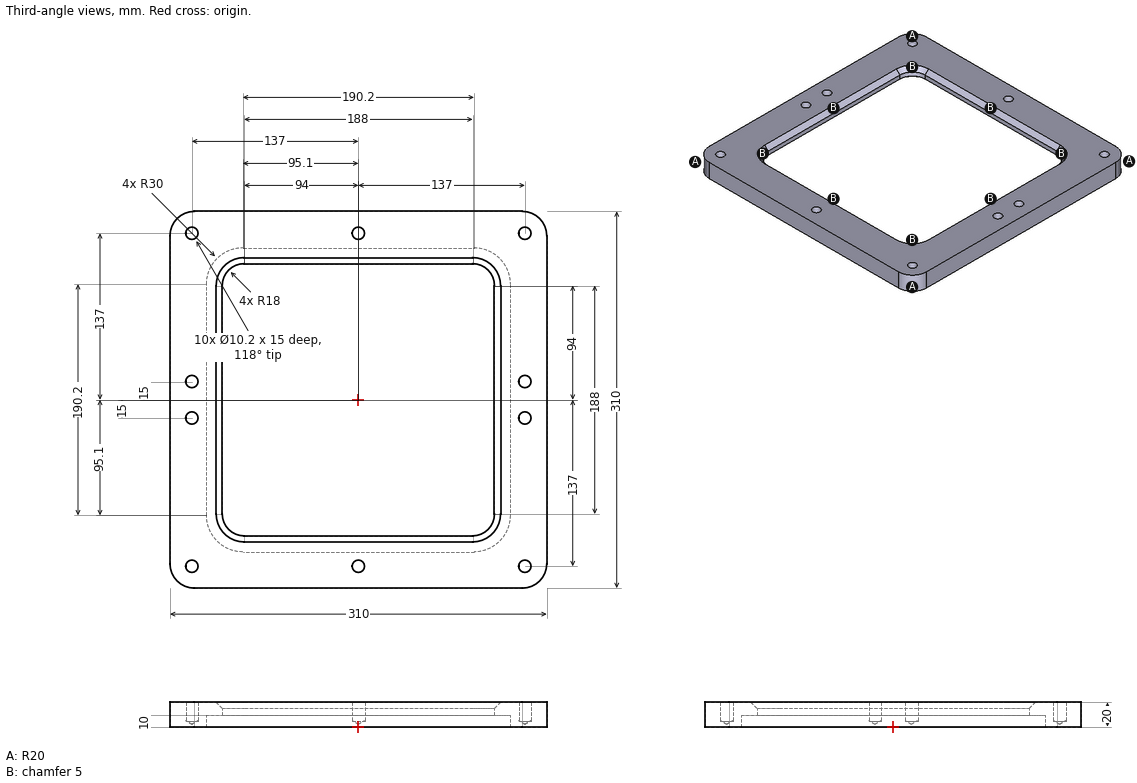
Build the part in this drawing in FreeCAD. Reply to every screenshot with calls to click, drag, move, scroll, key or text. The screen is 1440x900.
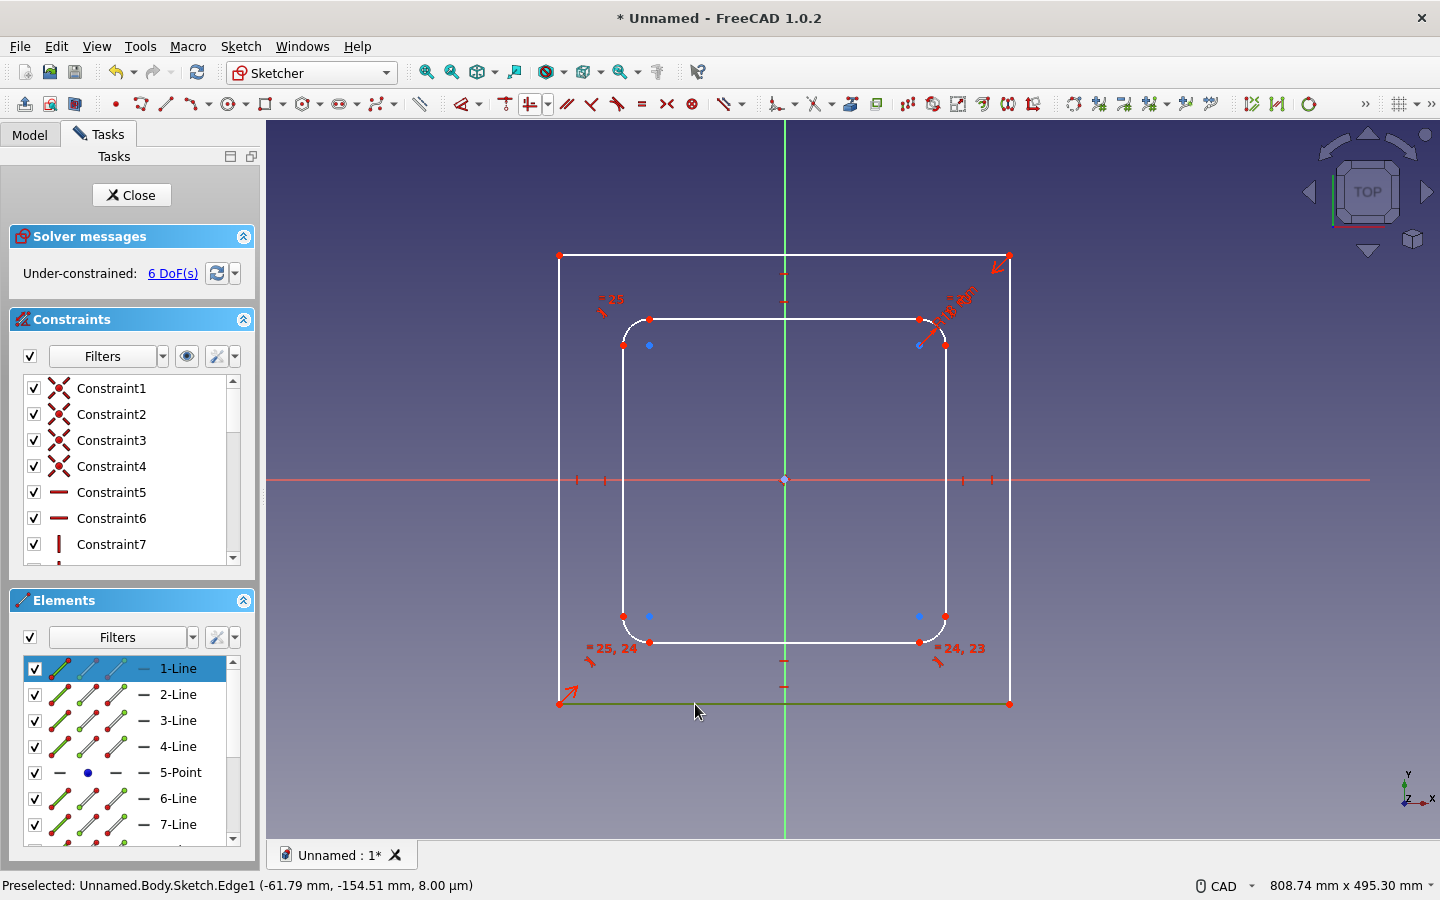
key(l)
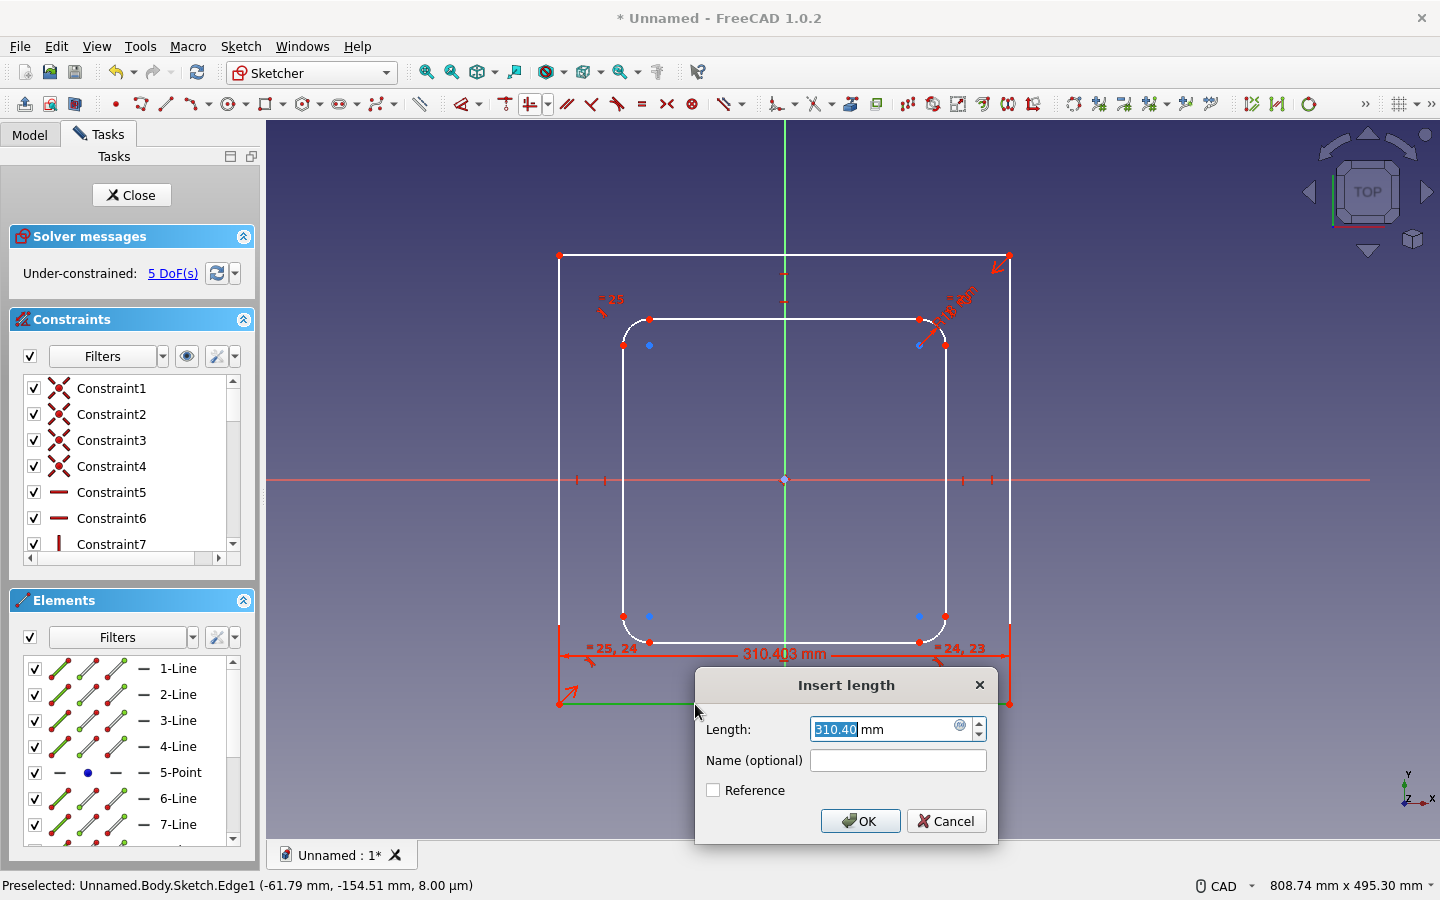
text(310)
key(Return)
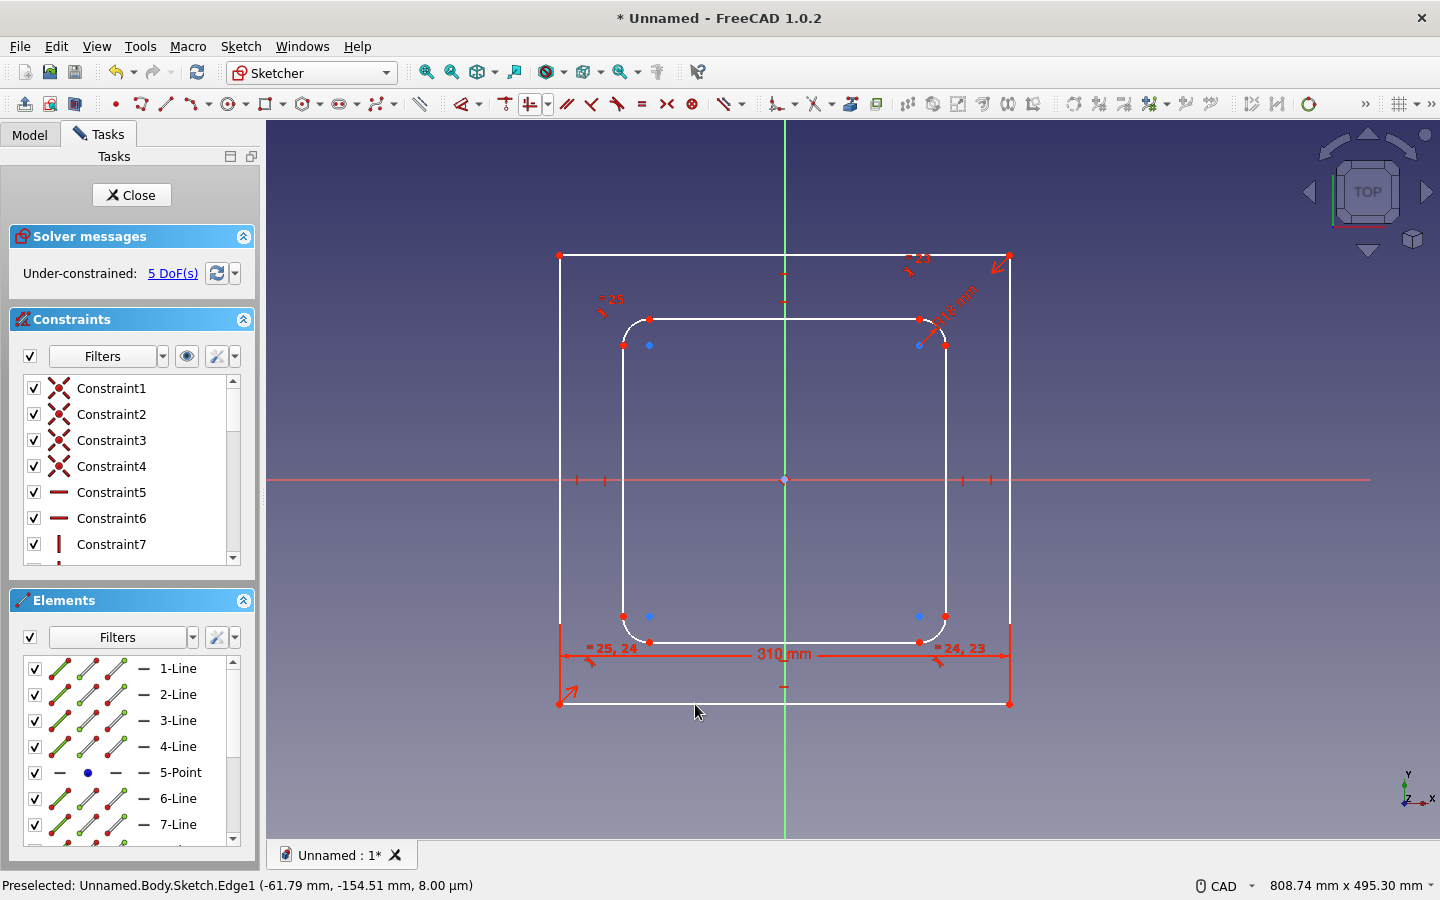
click(1010, 569)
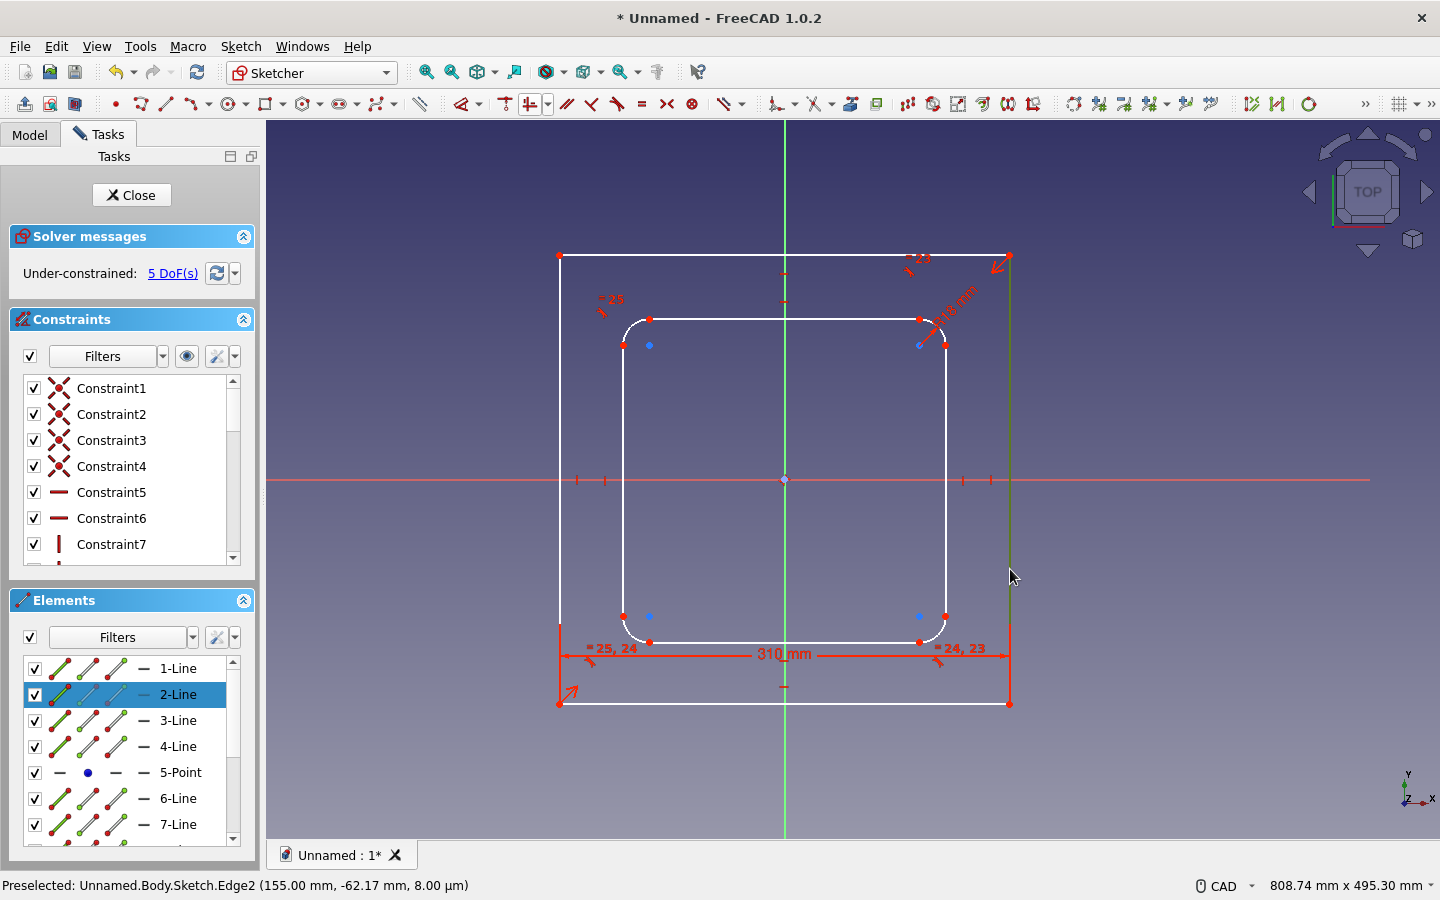
click(478, 104)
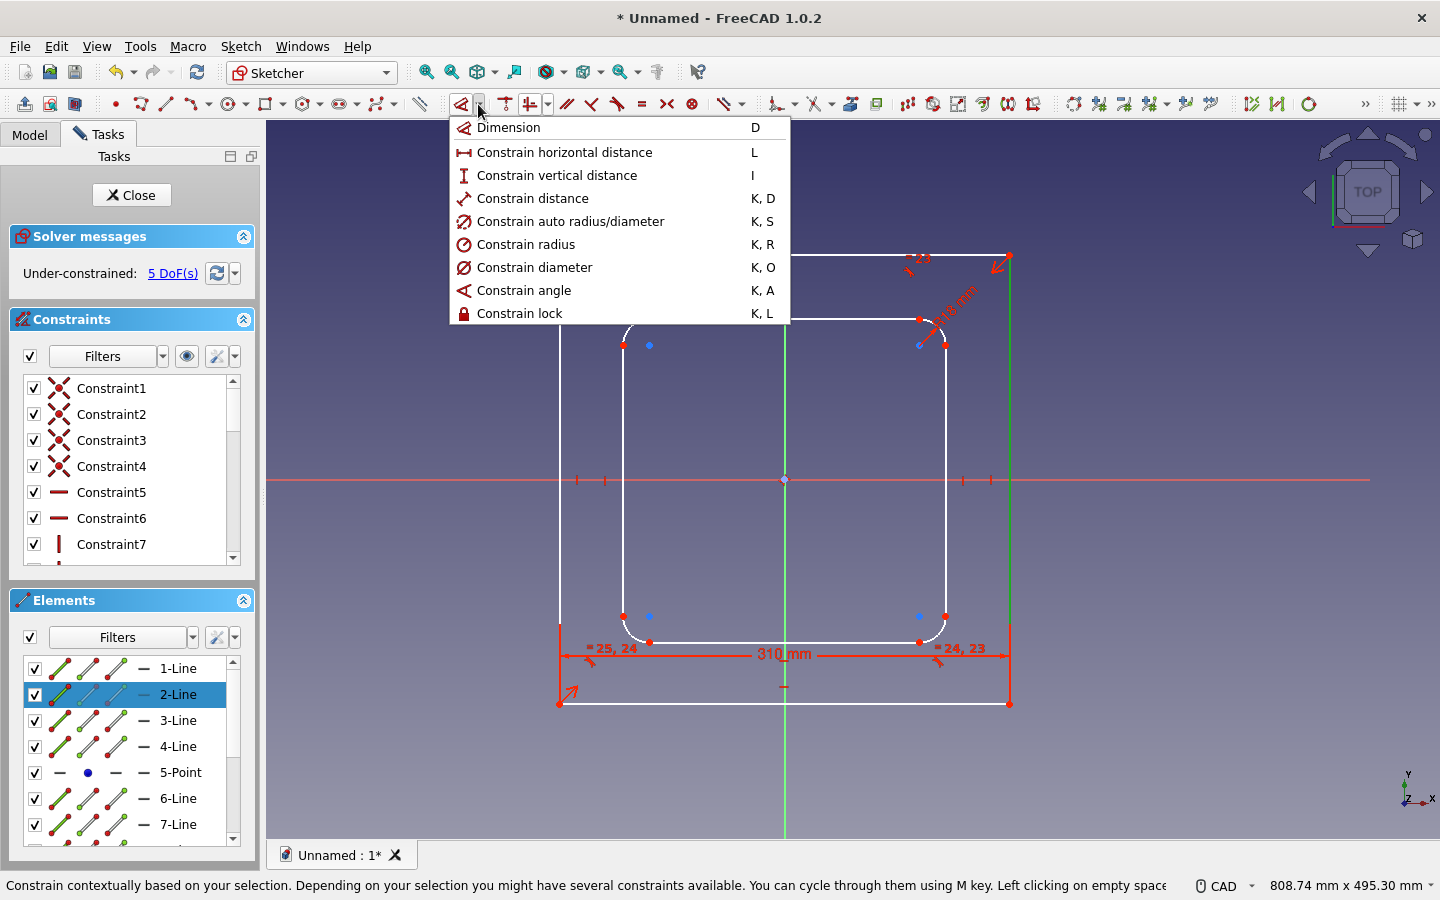
click(620, 176)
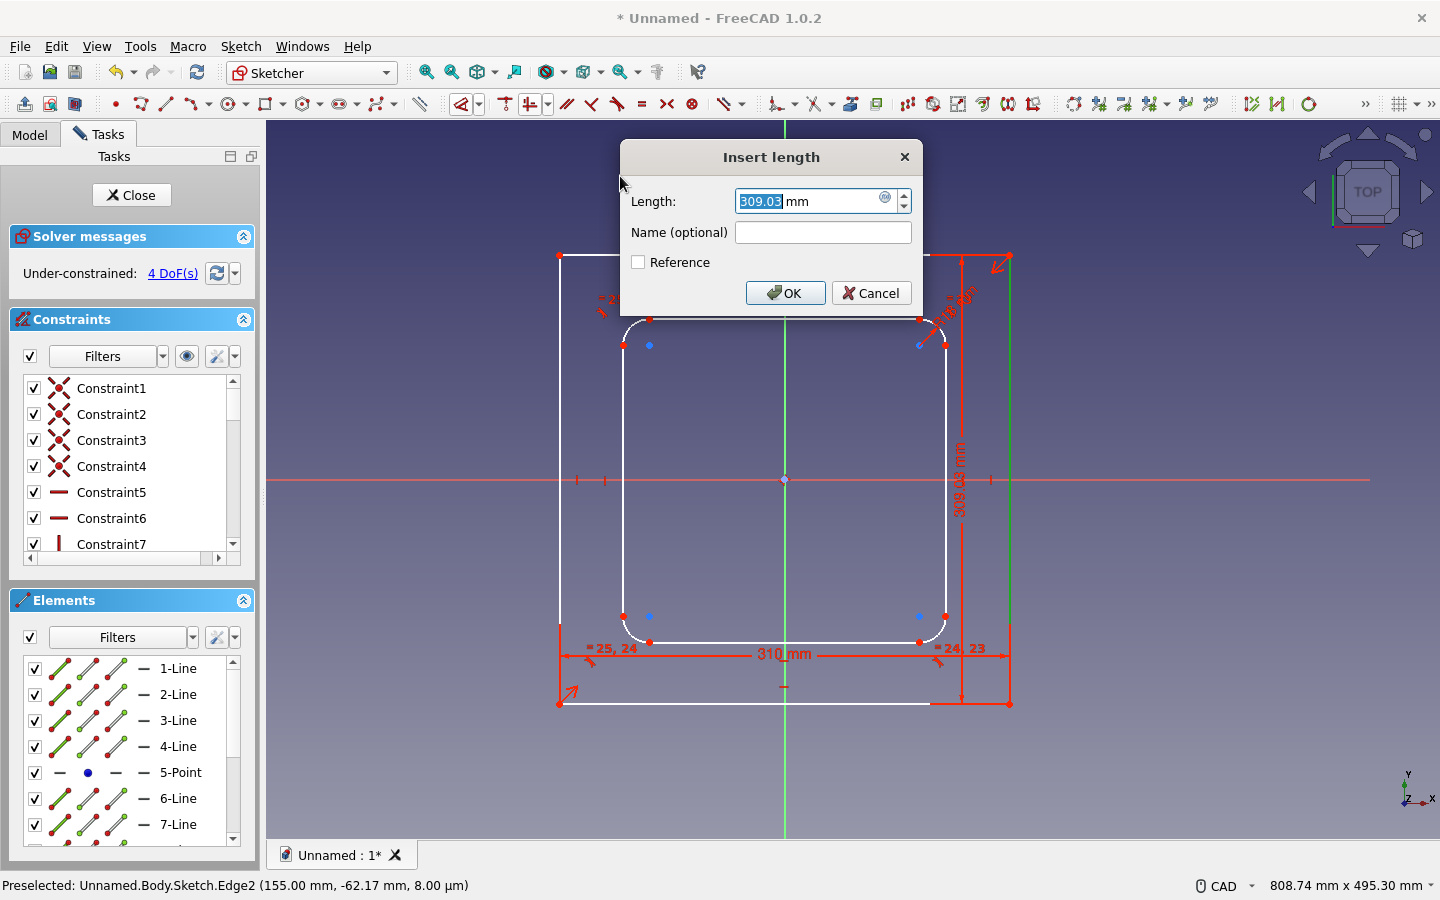
text(310)
key(Return)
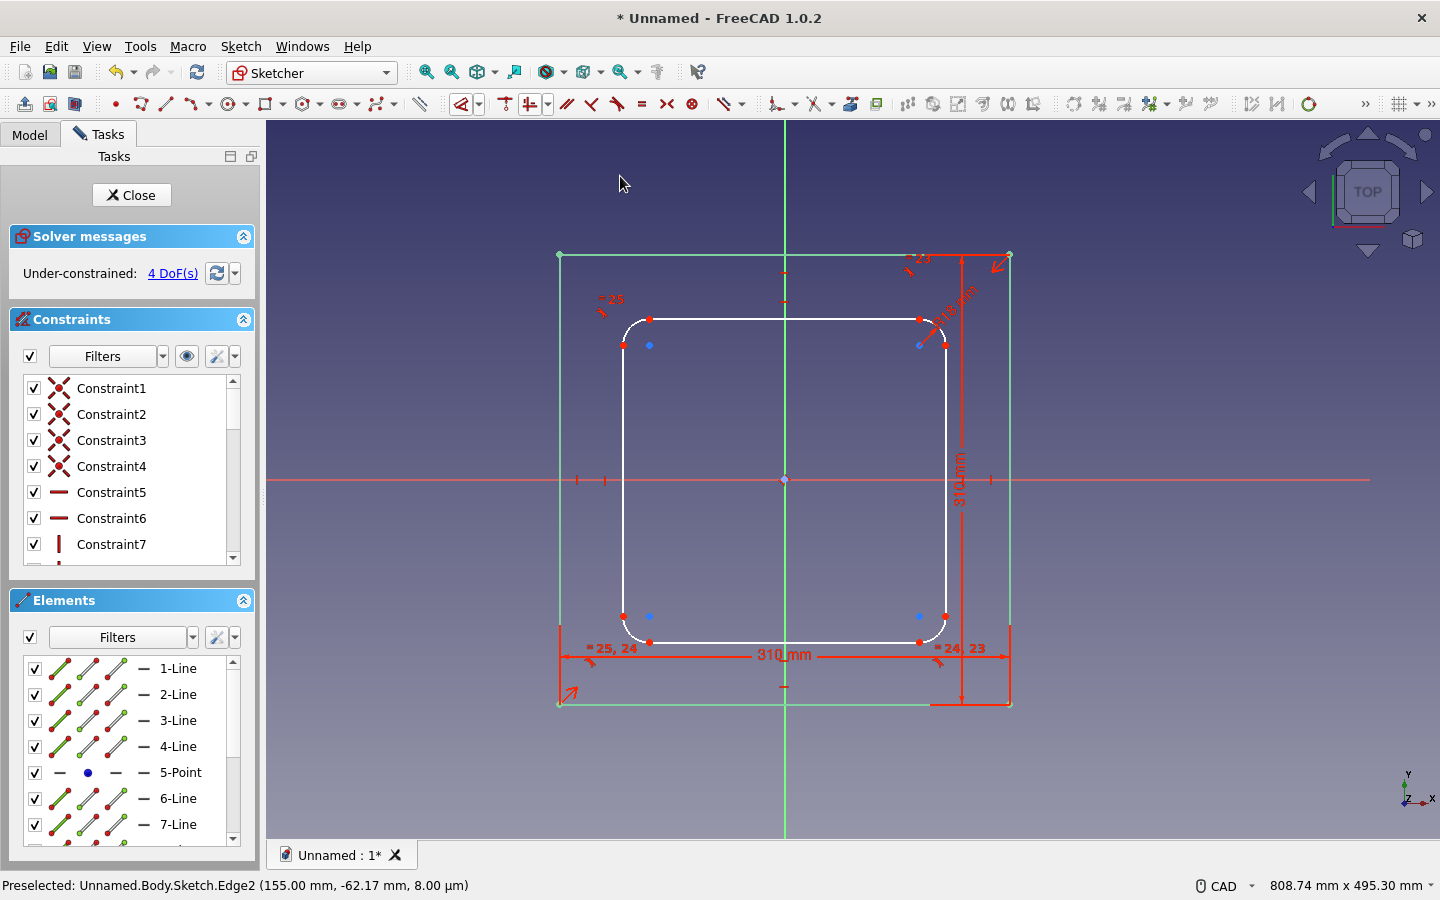
click(730, 319)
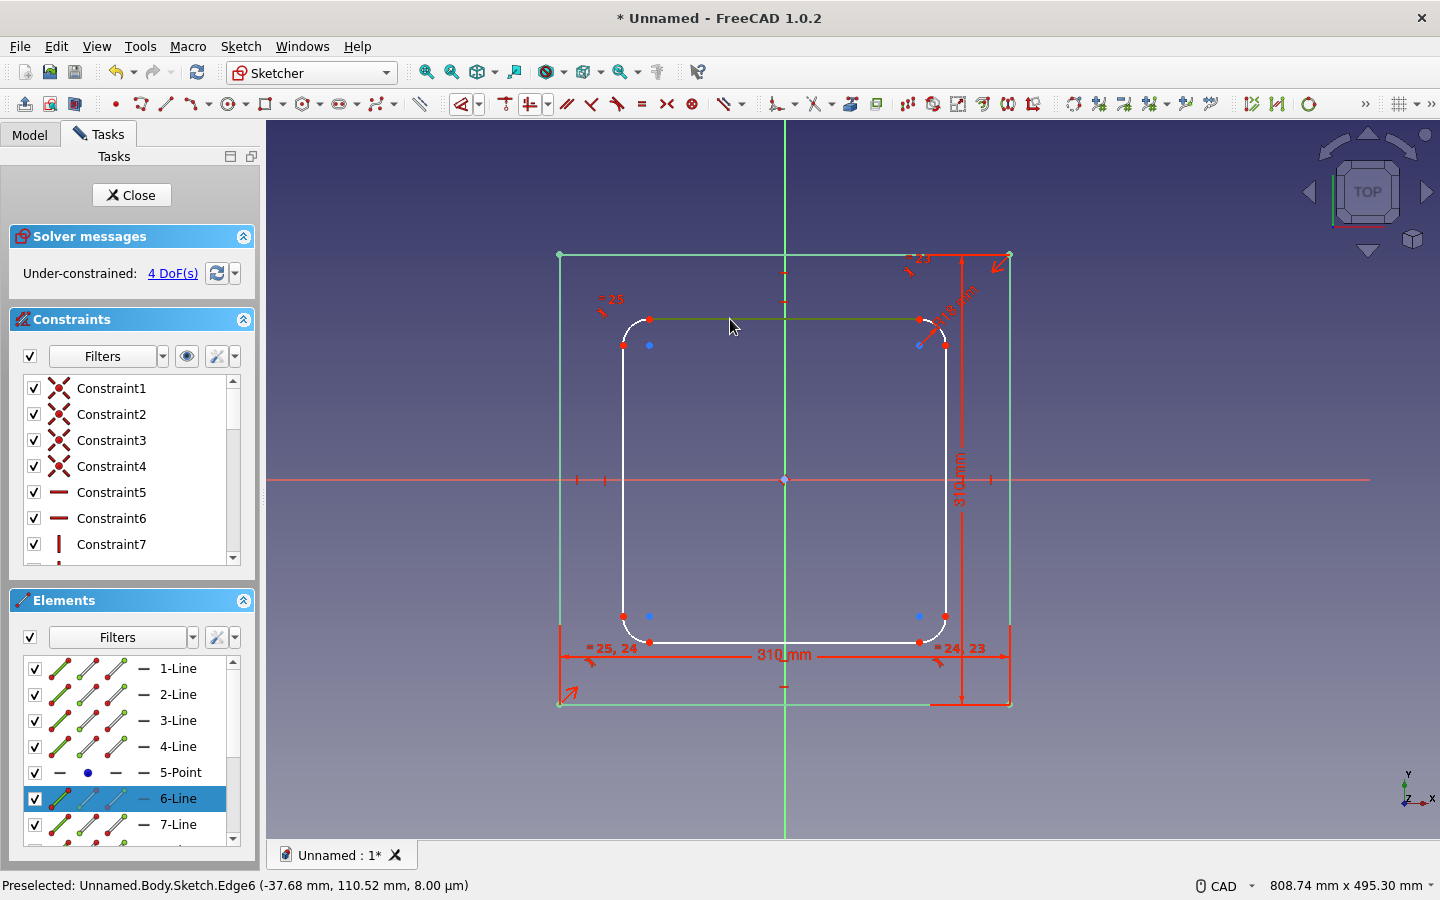
click(478, 104)